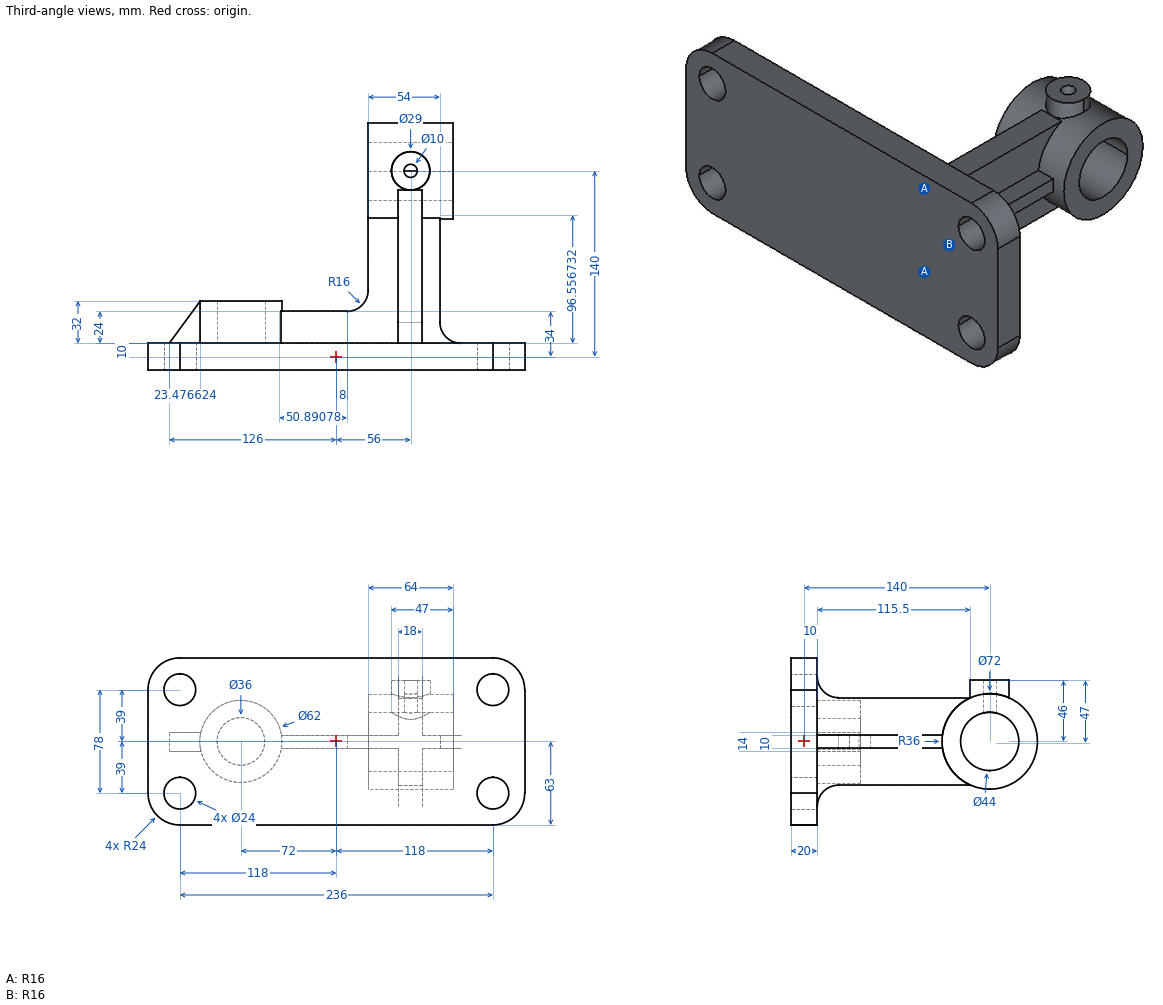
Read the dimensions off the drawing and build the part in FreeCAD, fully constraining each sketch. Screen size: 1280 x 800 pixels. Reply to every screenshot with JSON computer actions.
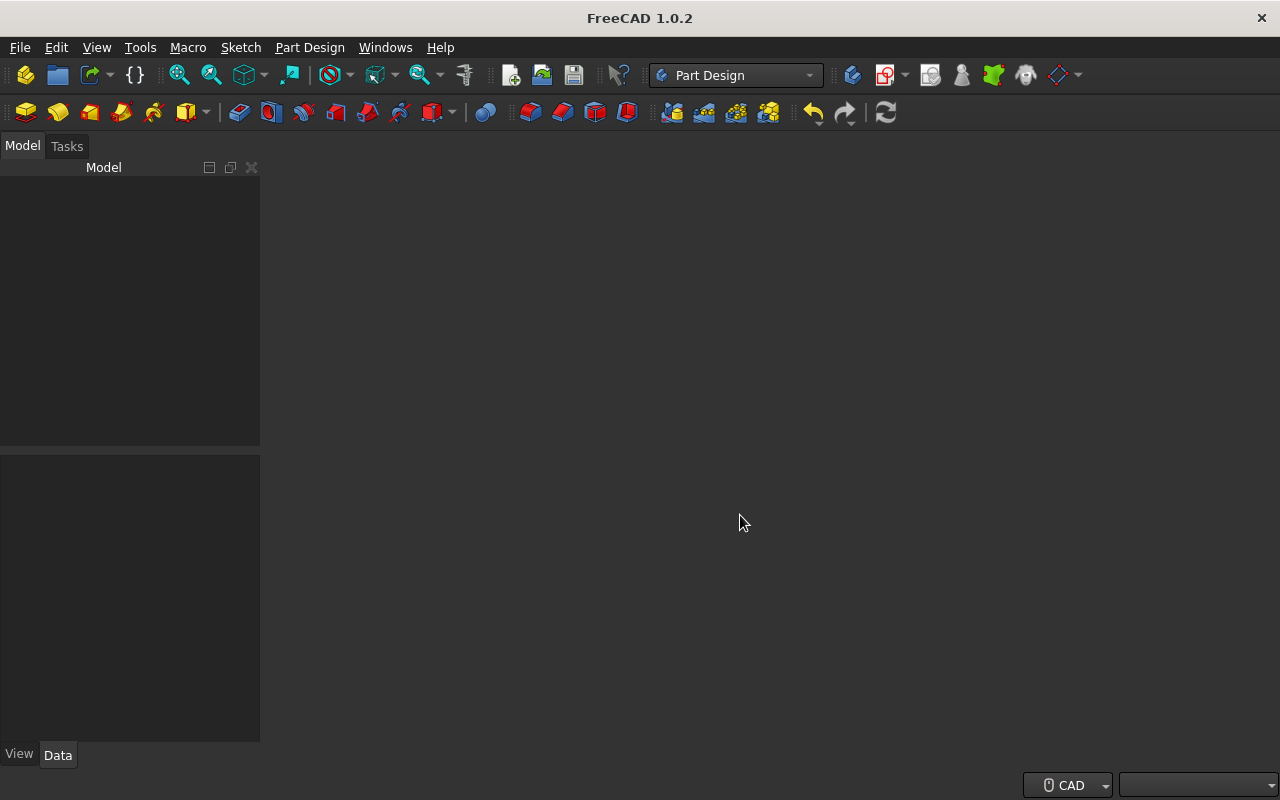
{"action": "left_click", "coordinate": [510, 76]}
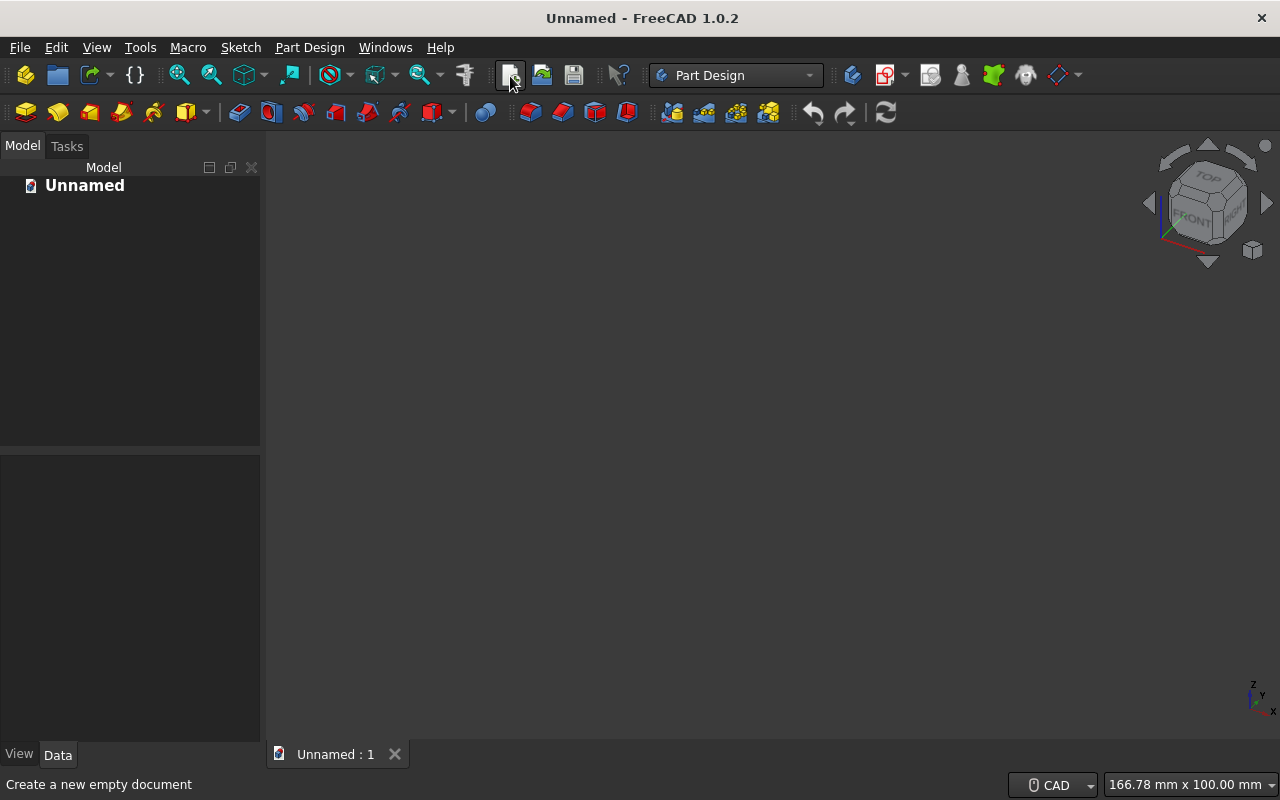
{"action": "left_click", "coordinate": [886, 76]}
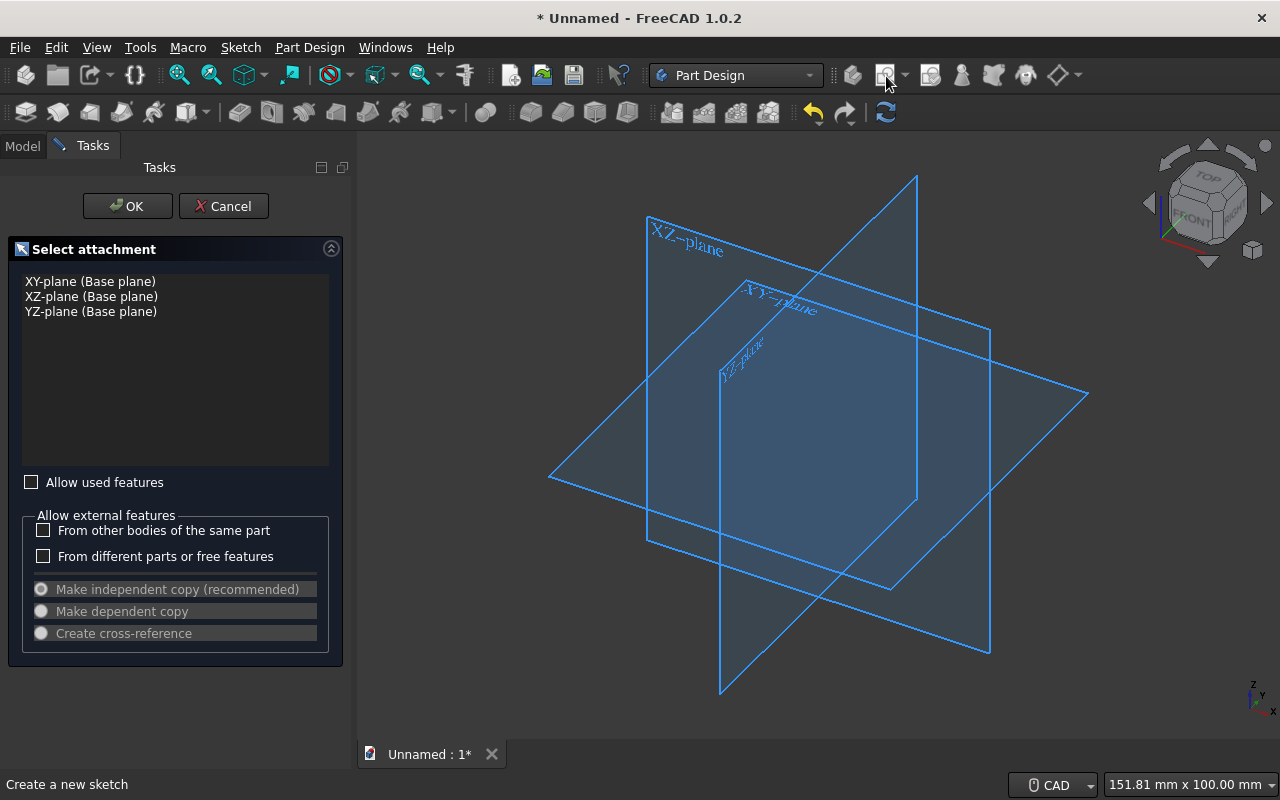
{"action": "left_click", "coordinate": [82, 296]}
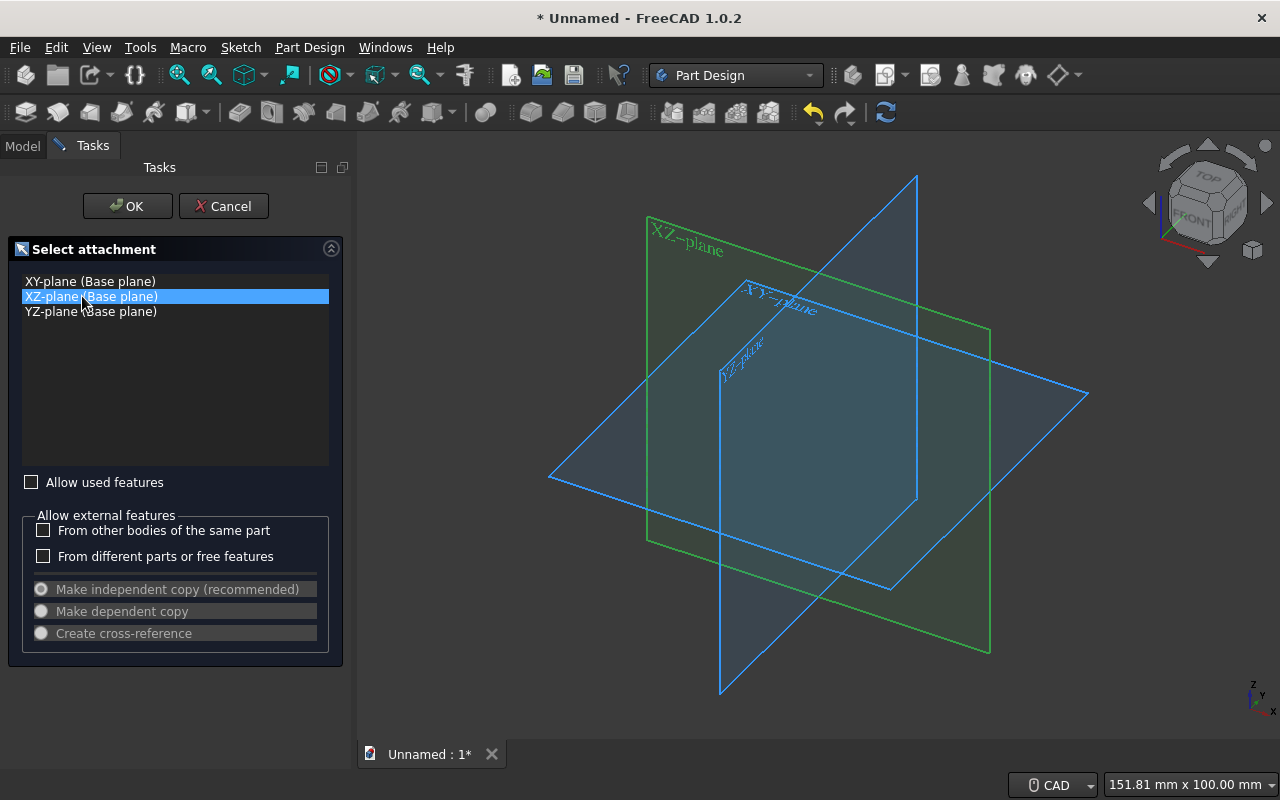
{"action": "left_click", "coordinate": [128, 206]}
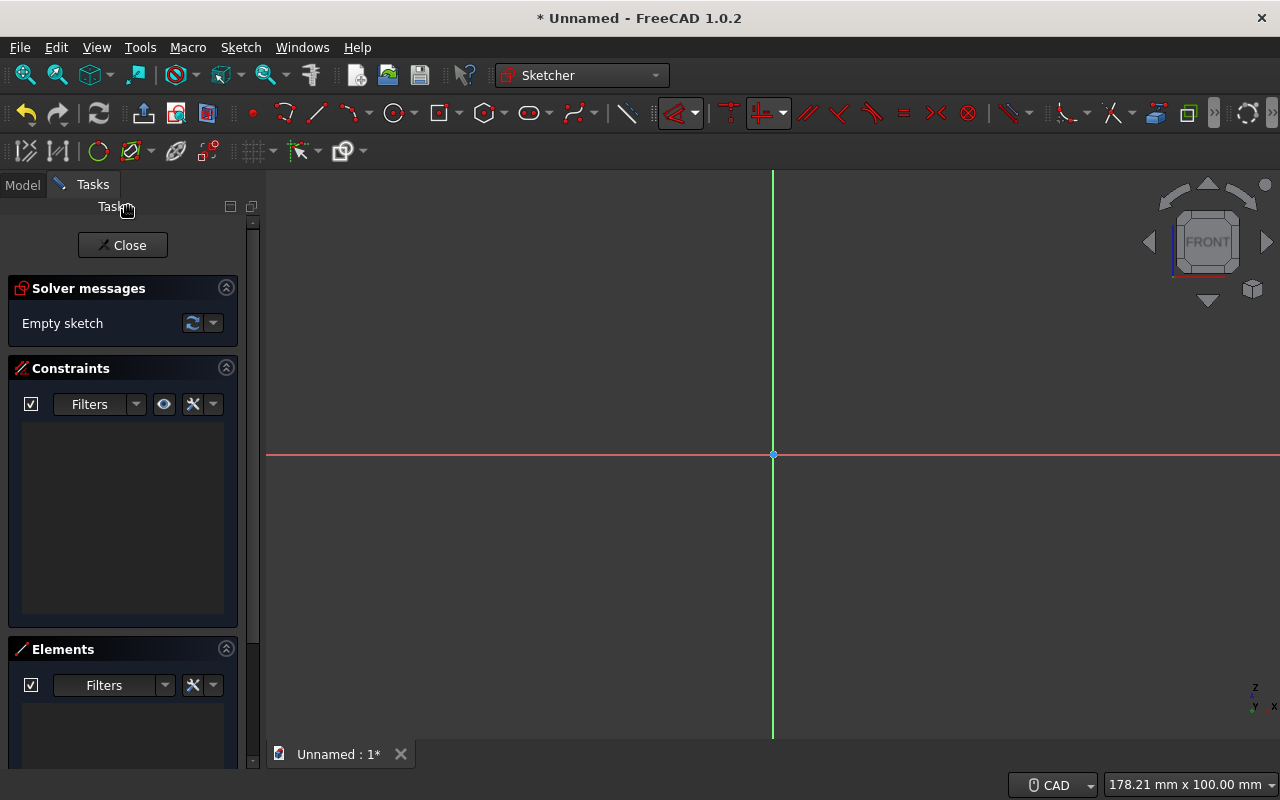
{"action": "scroll", "coordinate": [665, 454], "scroll_direction": "down", "scroll_amount": 5}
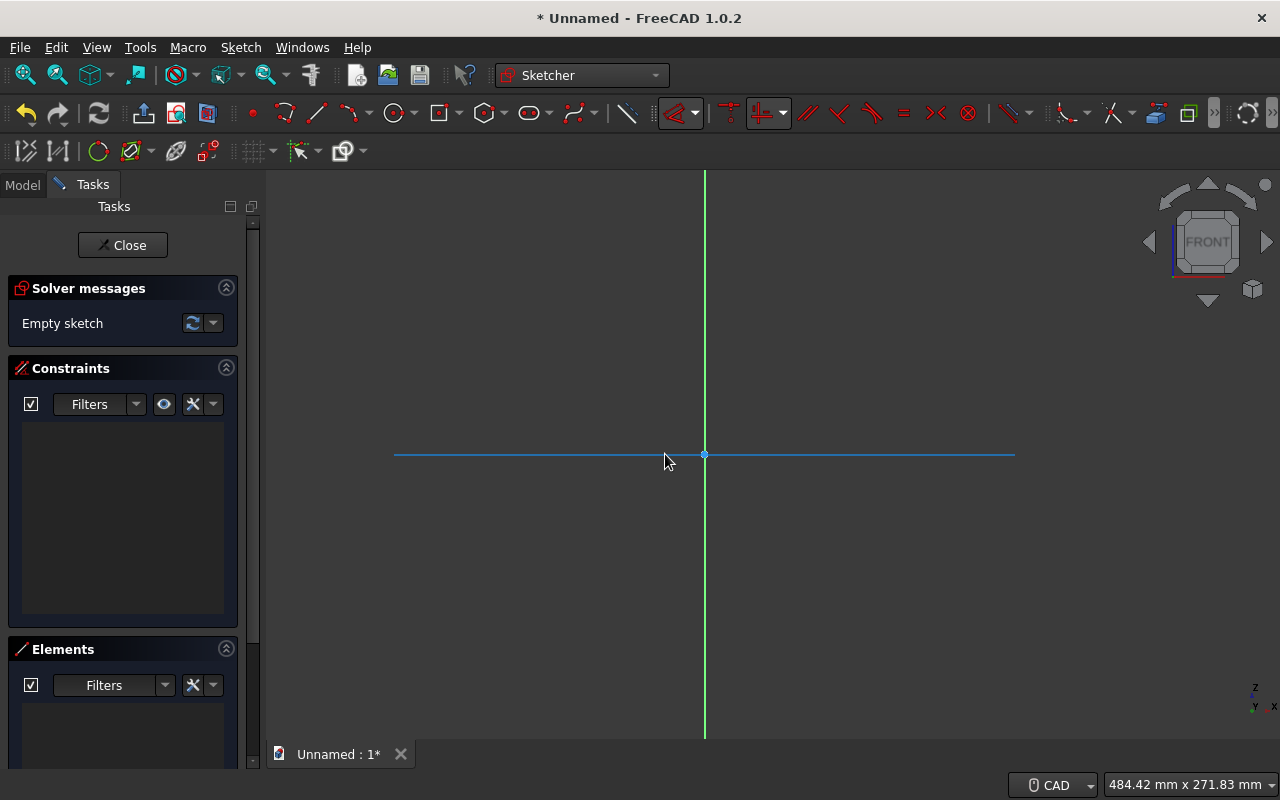
{"action": "left_click", "coordinate": [318, 114]}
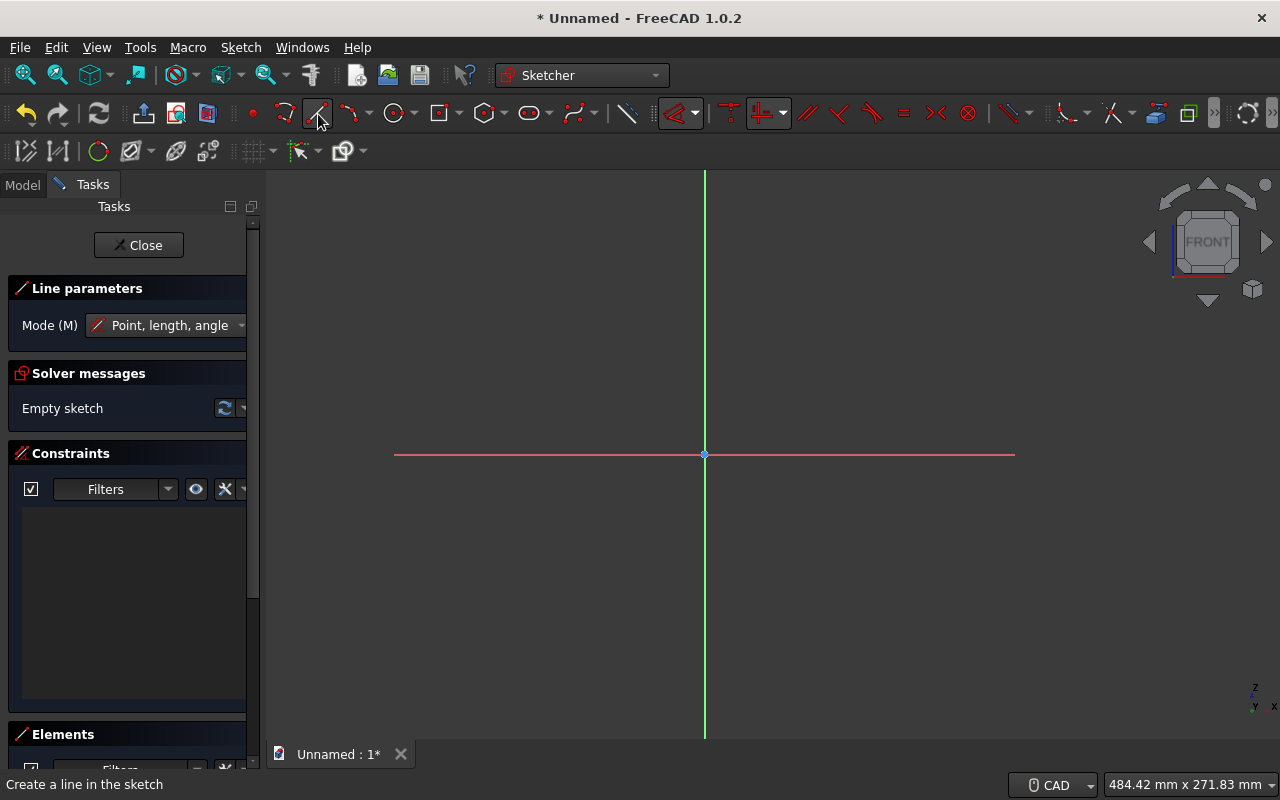
{"action": "left_click", "coordinate": [952, 586]}
{"action": "left_click", "coordinate": [458, 586]}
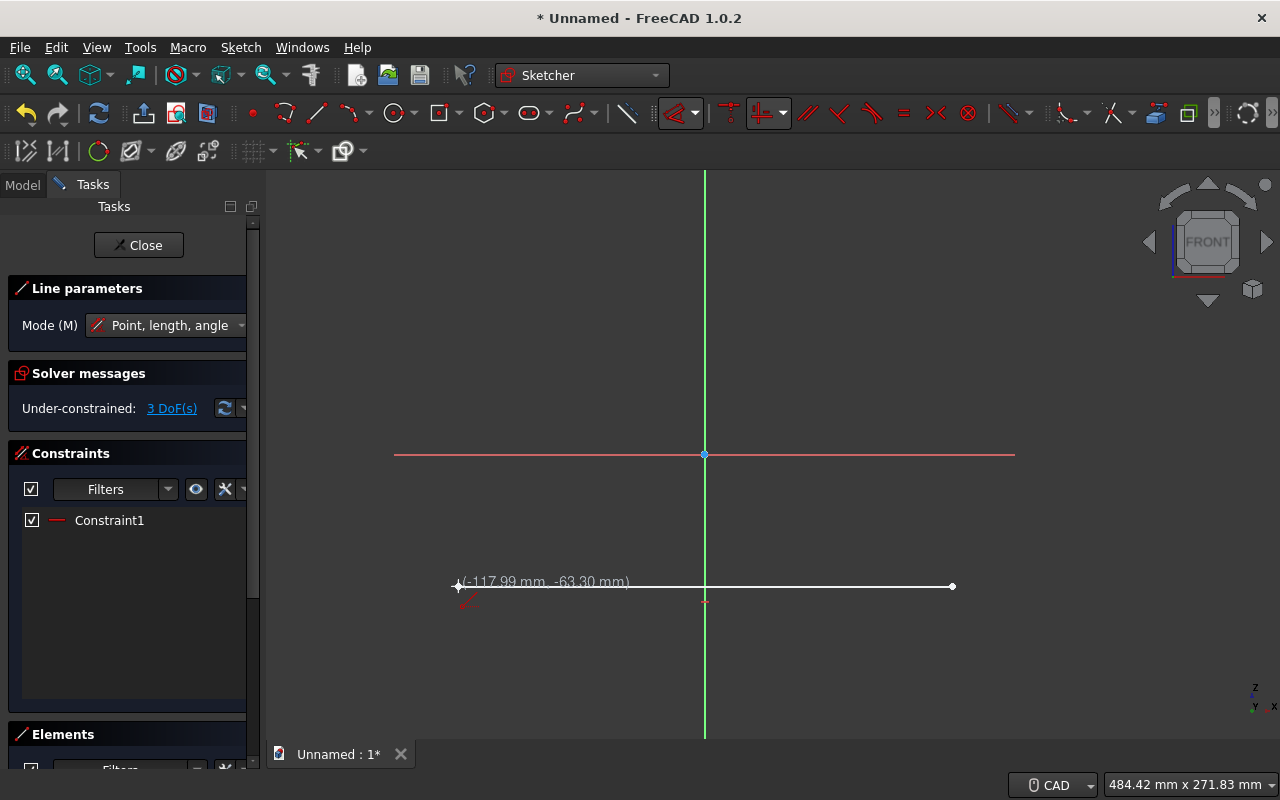
{"action": "left_click", "coordinate": [408, 536]}
{"action": "left_click", "coordinate": [408, 373]}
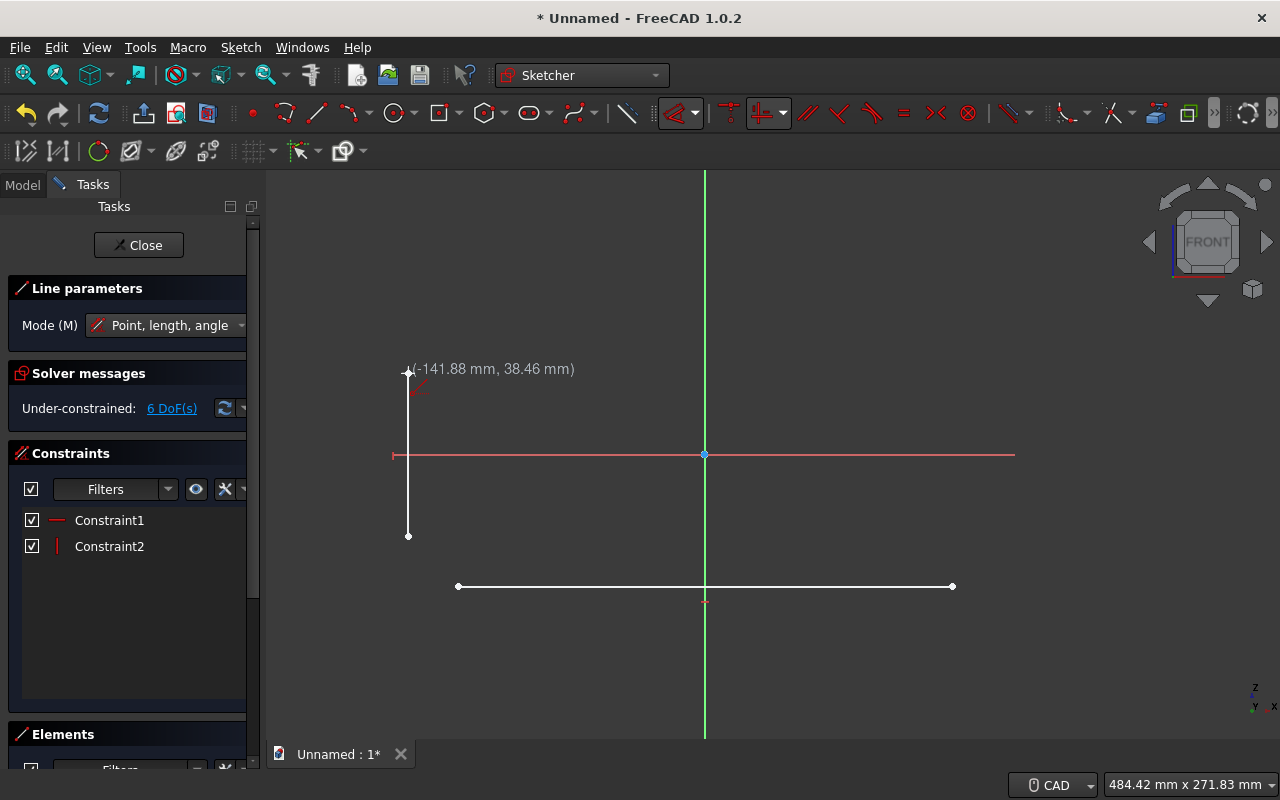
{"action": "left_click", "coordinate": [458, 323]}
{"action": "left_click", "coordinate": [952, 323]}